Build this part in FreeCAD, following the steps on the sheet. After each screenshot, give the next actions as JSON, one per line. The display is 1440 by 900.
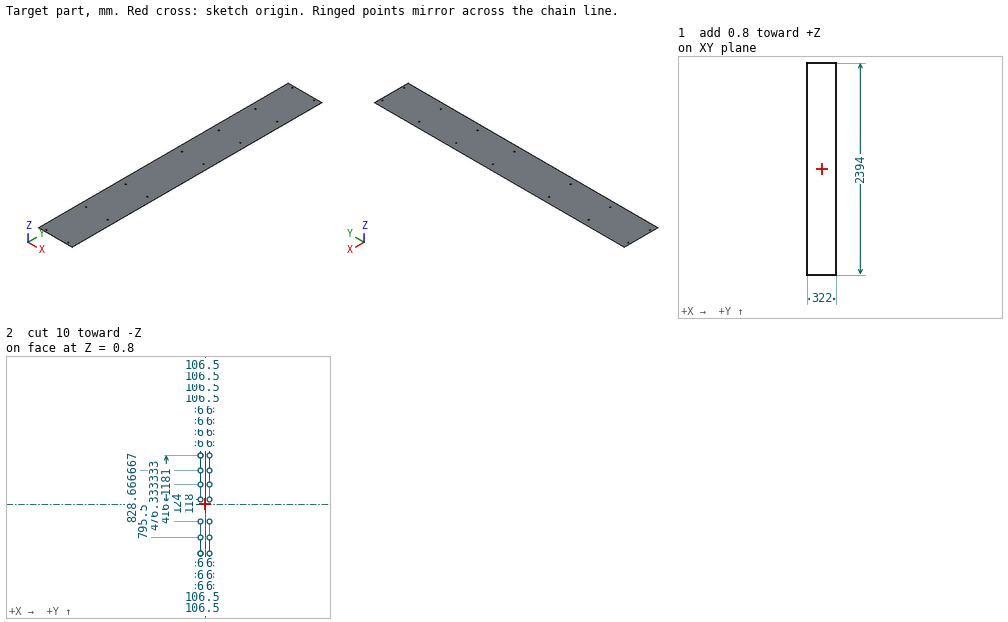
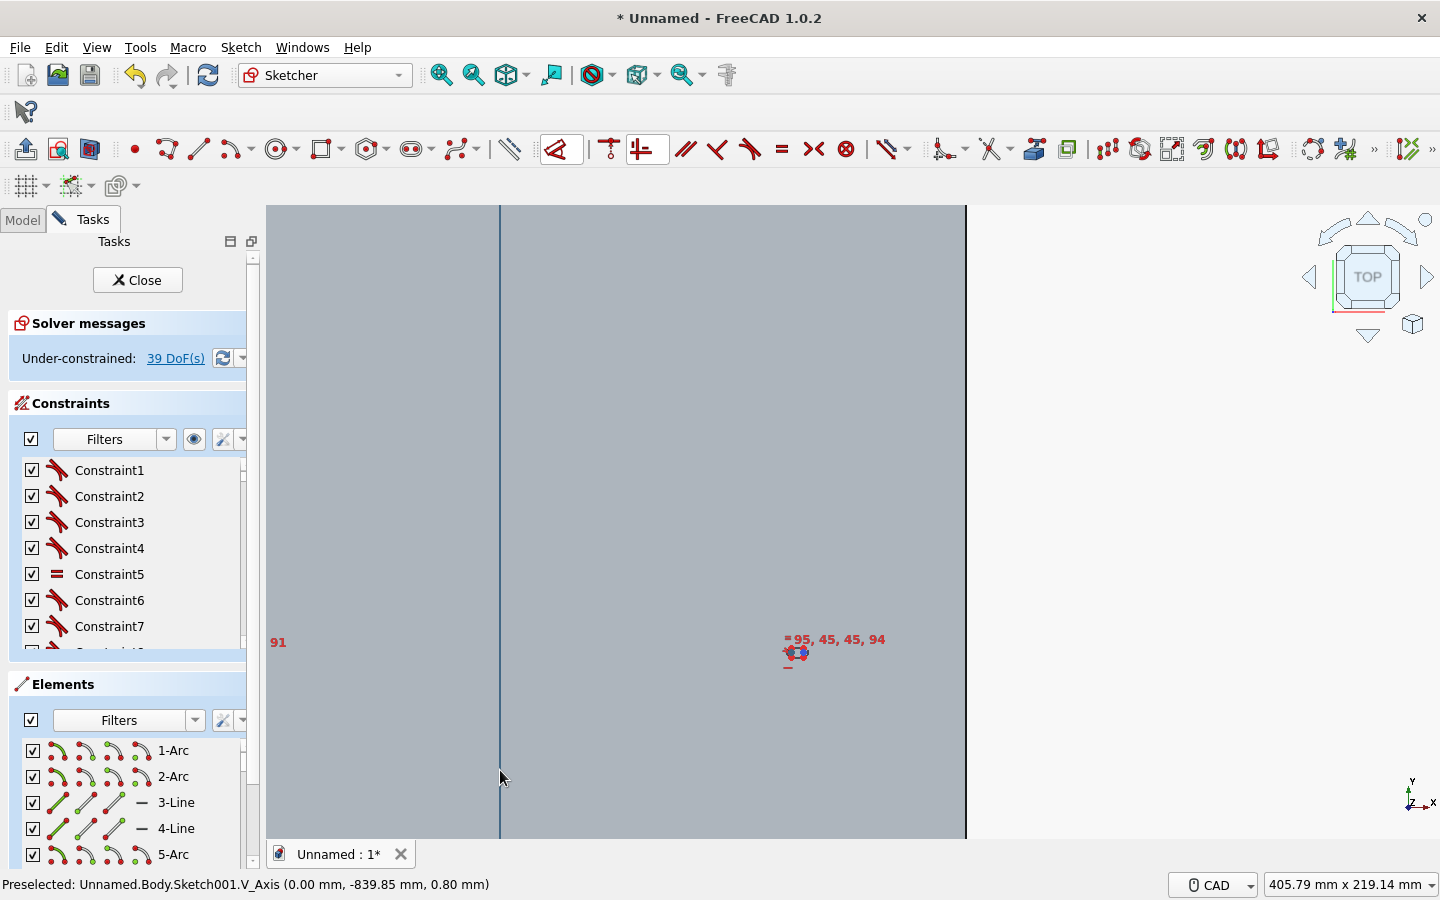
{"action": "left_click", "coordinate": [814, 150]}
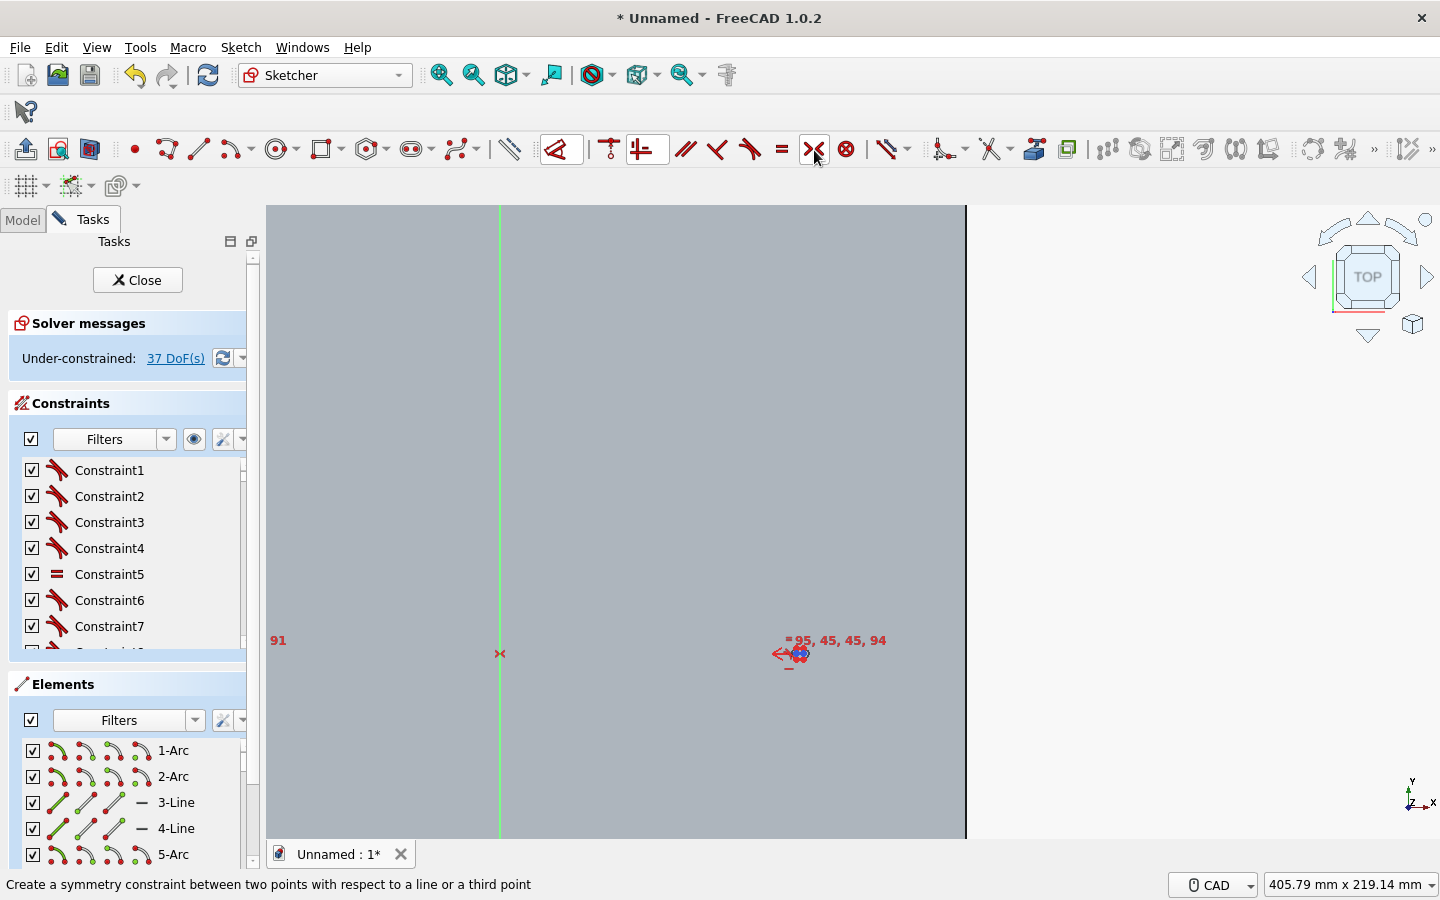
{"action": "scroll", "coordinate": [803, 663], "scroll_direction": "down", "scroll_amount": 14}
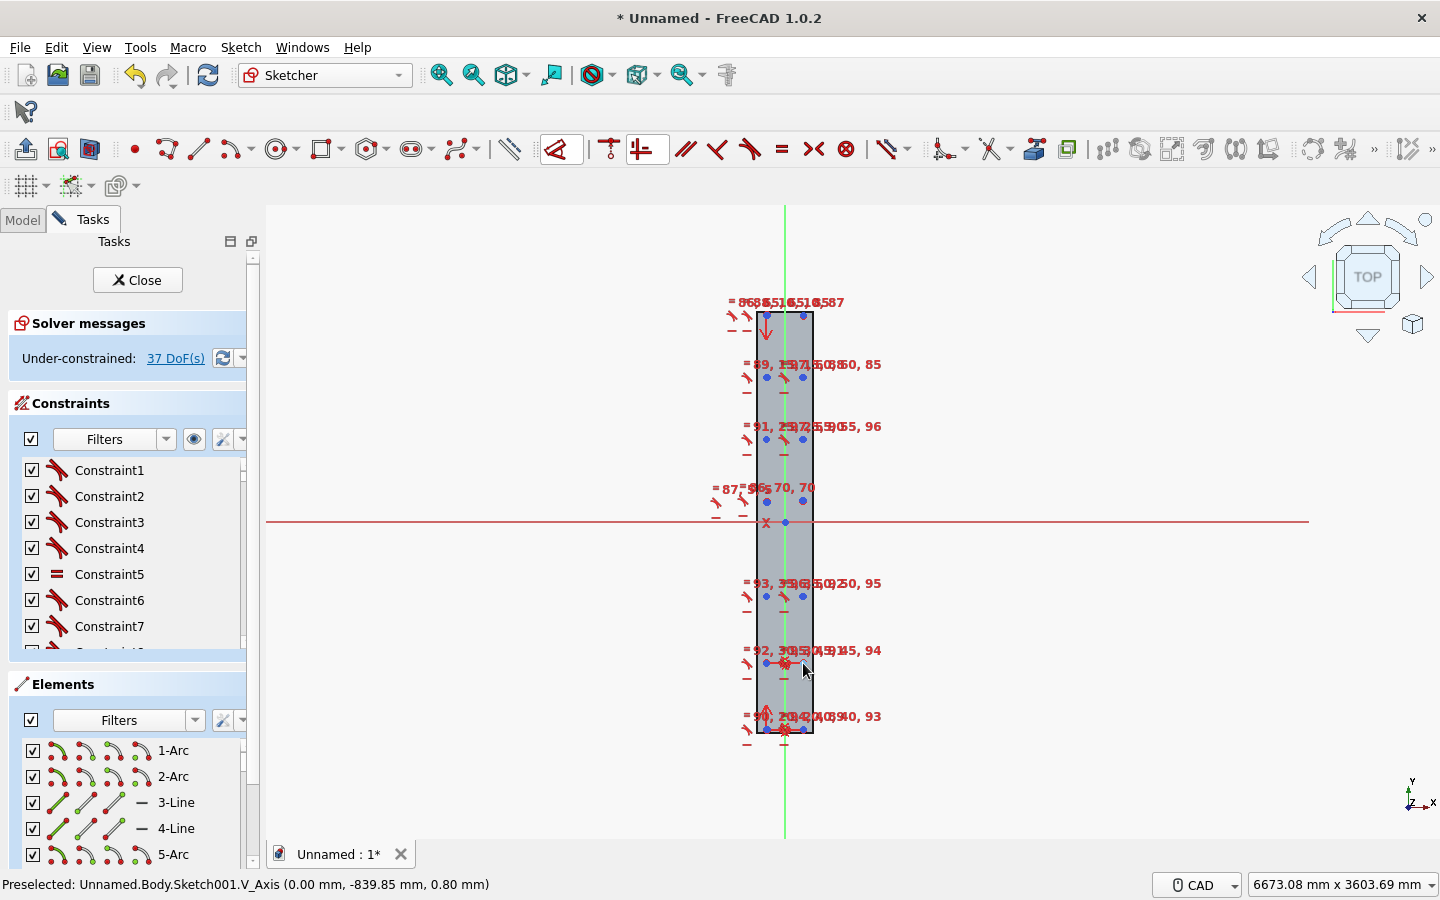
{"action": "scroll", "coordinate": [767, 597], "scroll_direction": "up", "scroll_amount": 14}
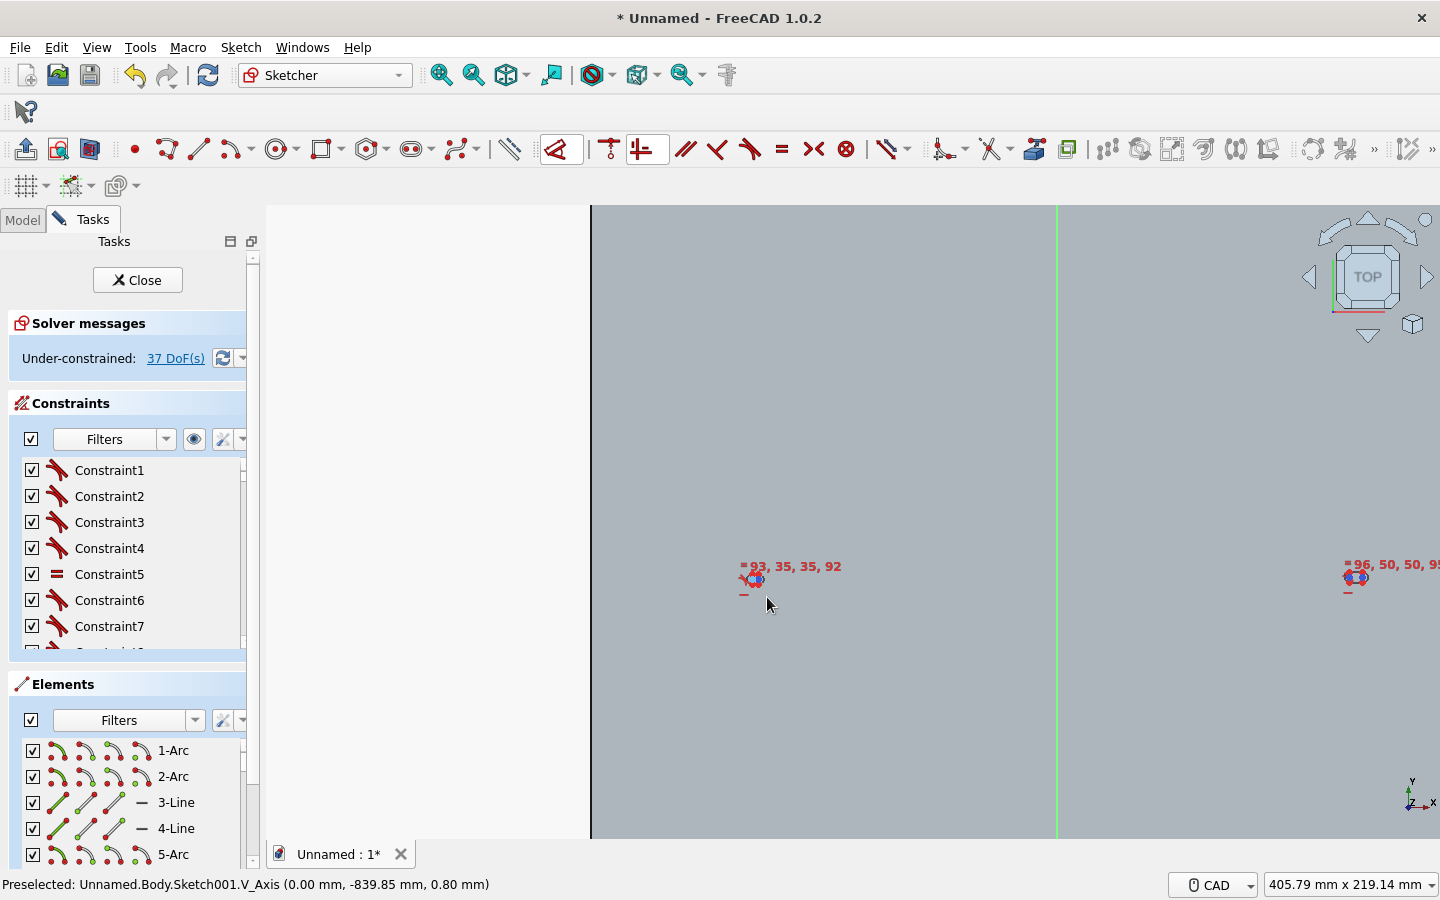
{"action": "left_click", "coordinate": [758, 579]}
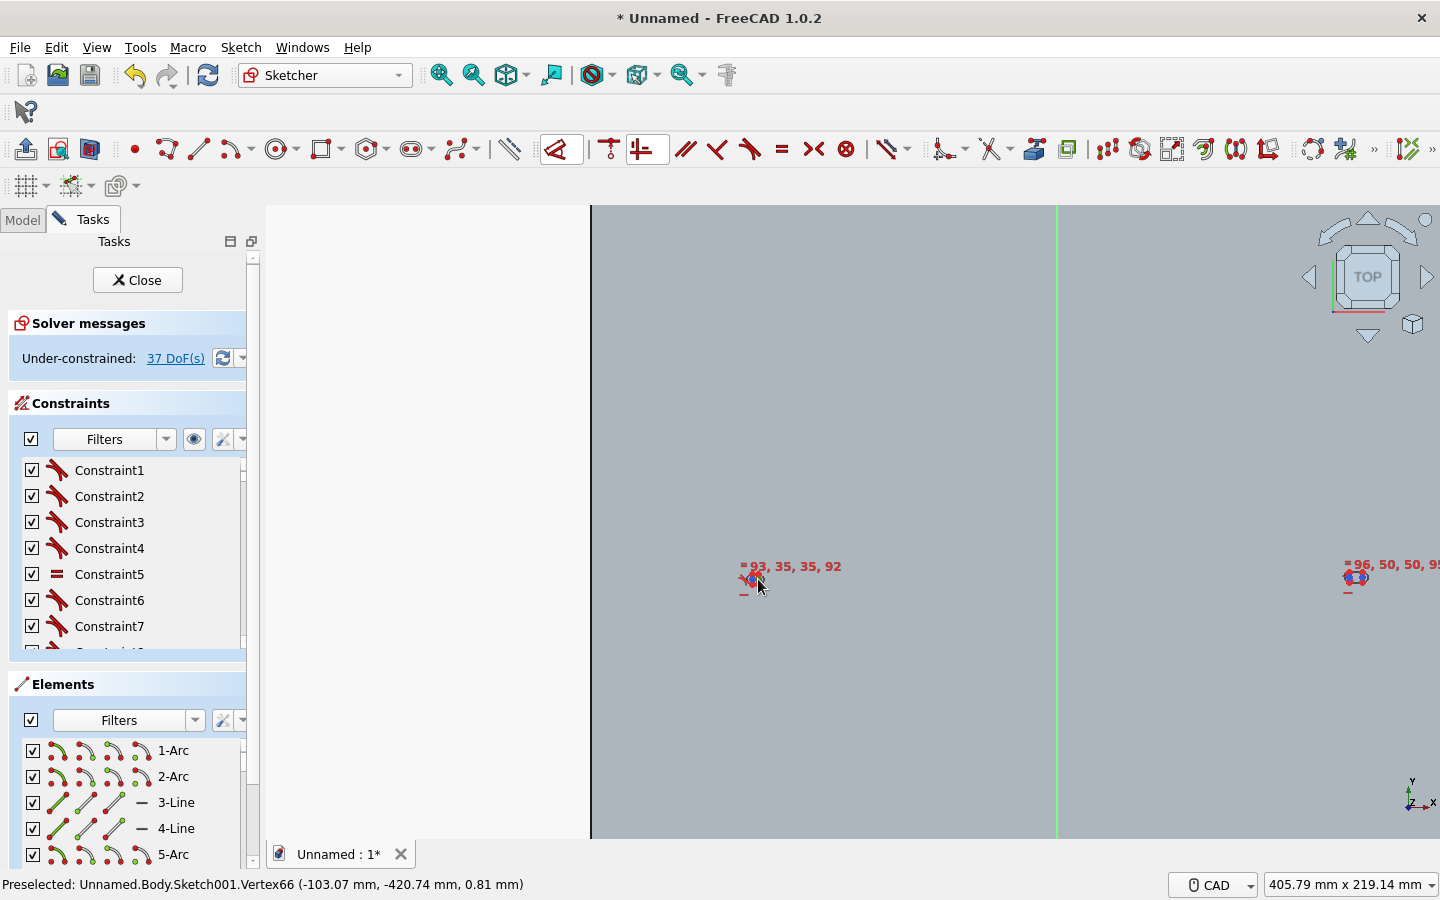
{"action": "scroll", "coordinate": [767, 597], "scroll_direction": "down", "scroll_amount": 14}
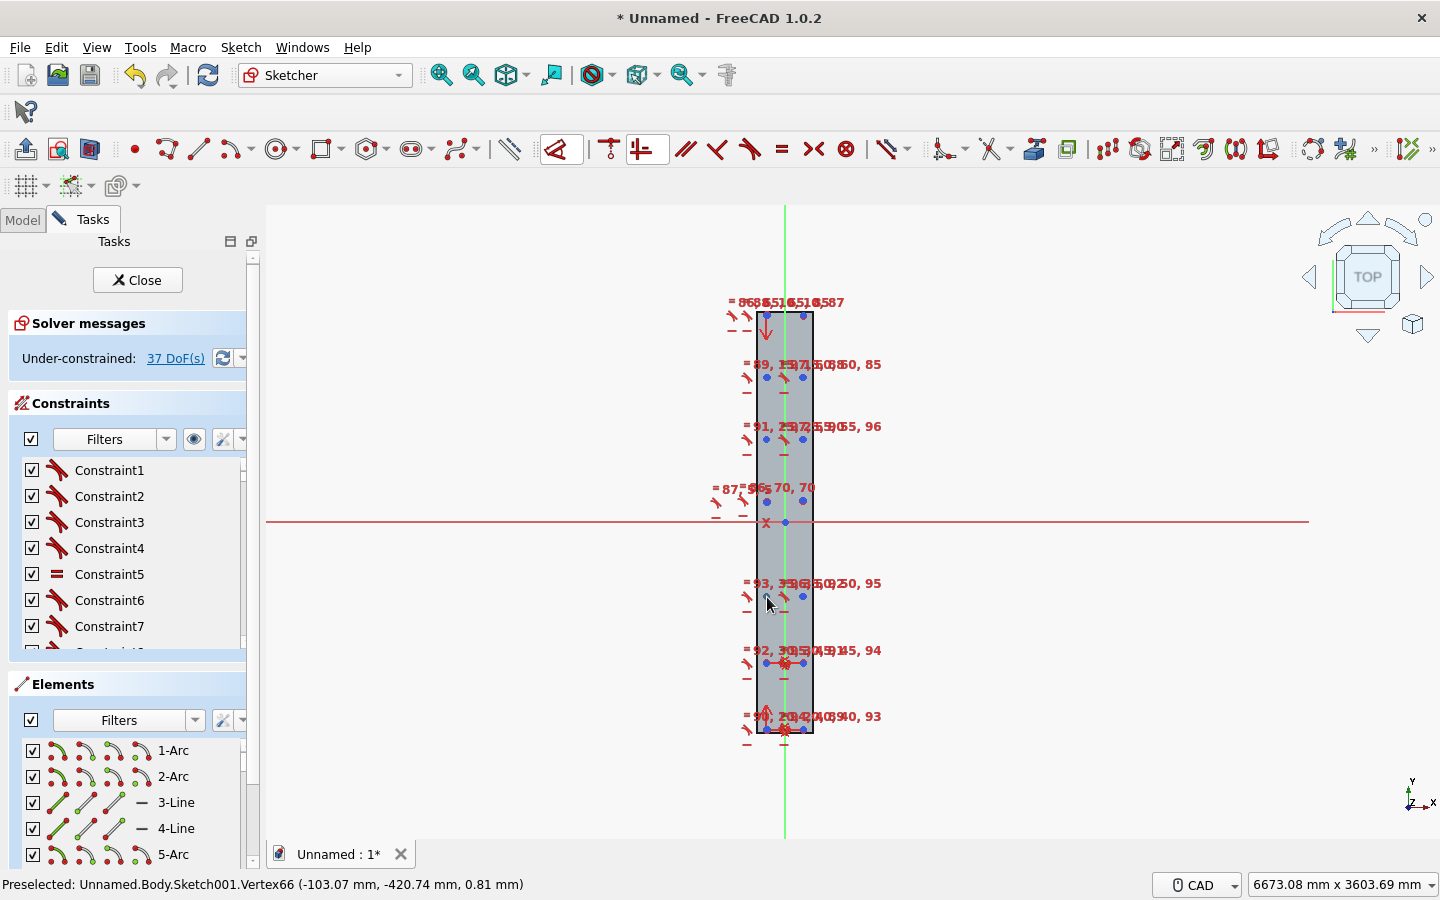
{"action": "scroll", "coordinate": [803, 596], "scroll_direction": "up", "scroll_amount": 14}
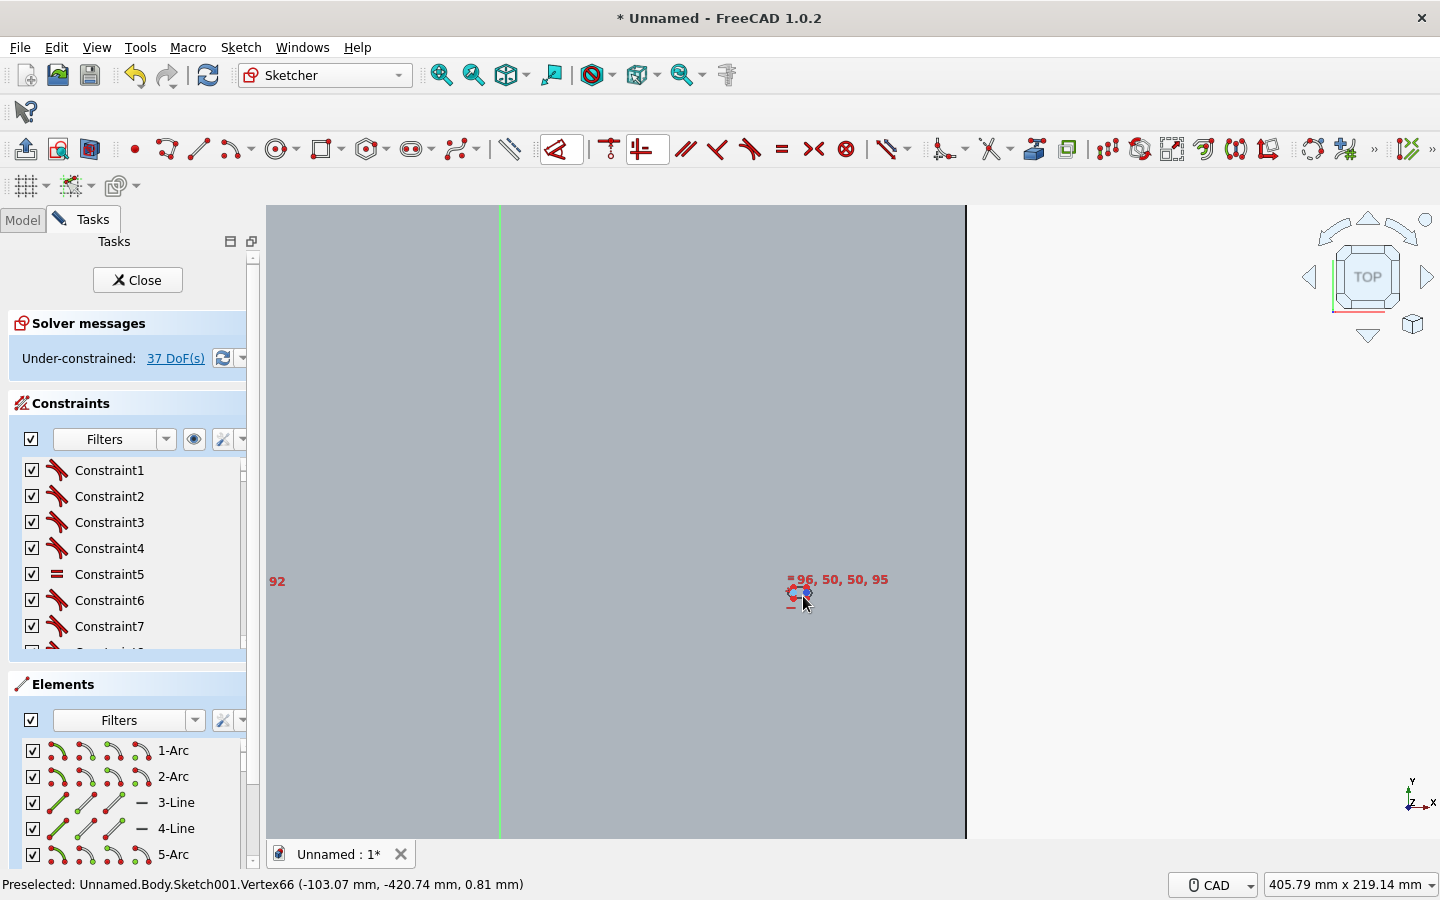
{"action": "left_click", "coordinate": [793, 593]}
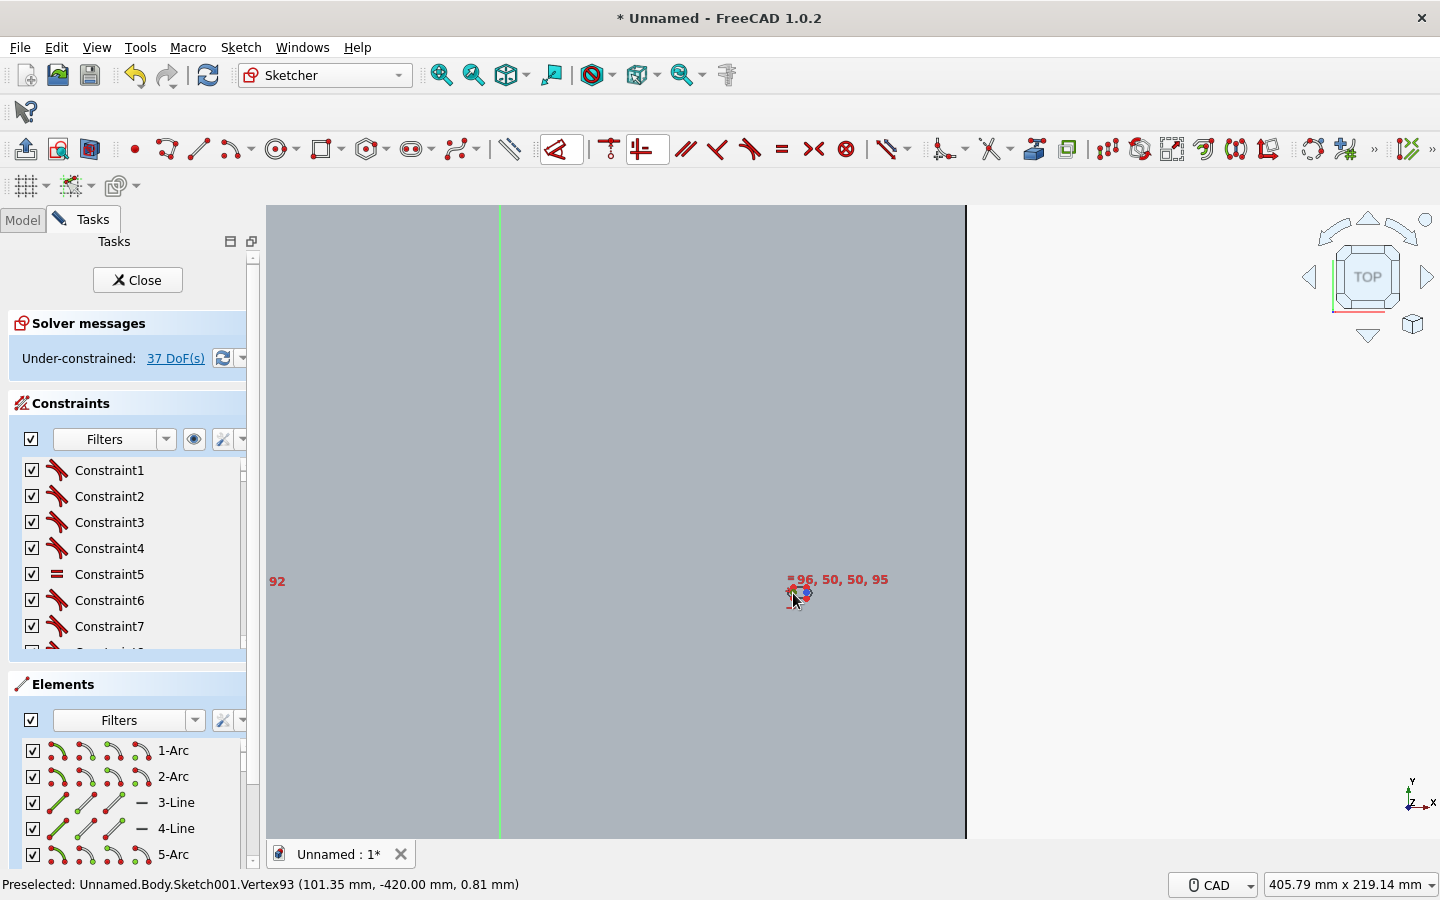
{"action": "left_click", "coordinate": [500, 770]}